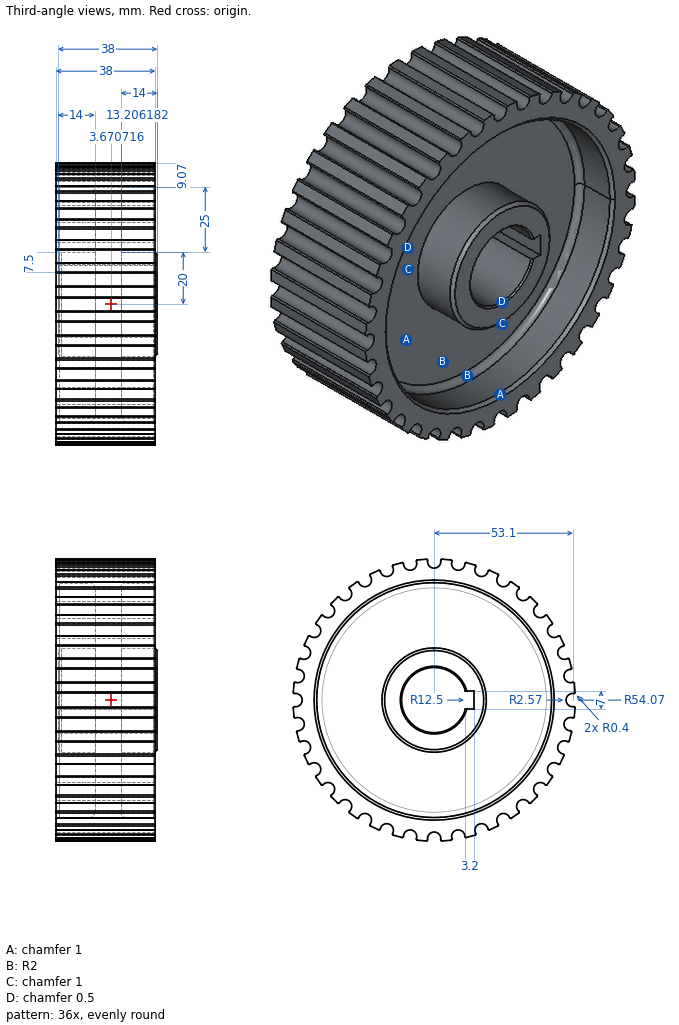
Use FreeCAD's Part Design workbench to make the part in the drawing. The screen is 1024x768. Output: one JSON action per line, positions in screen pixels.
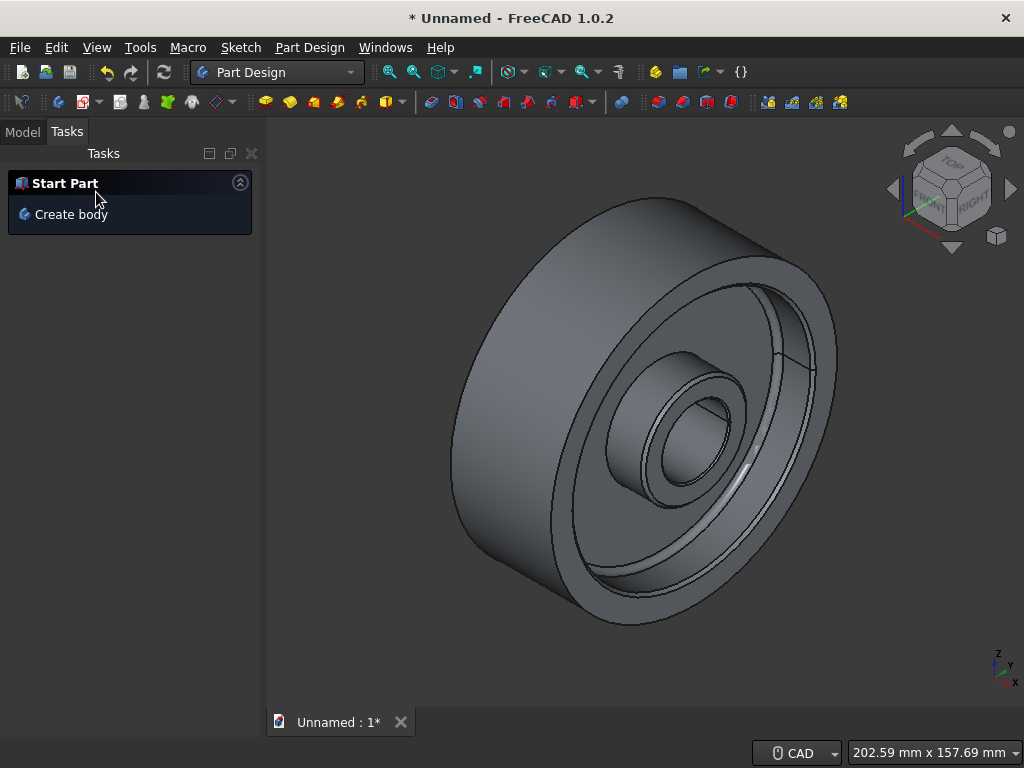
{"action": "left_click", "coordinate": [739, 416]}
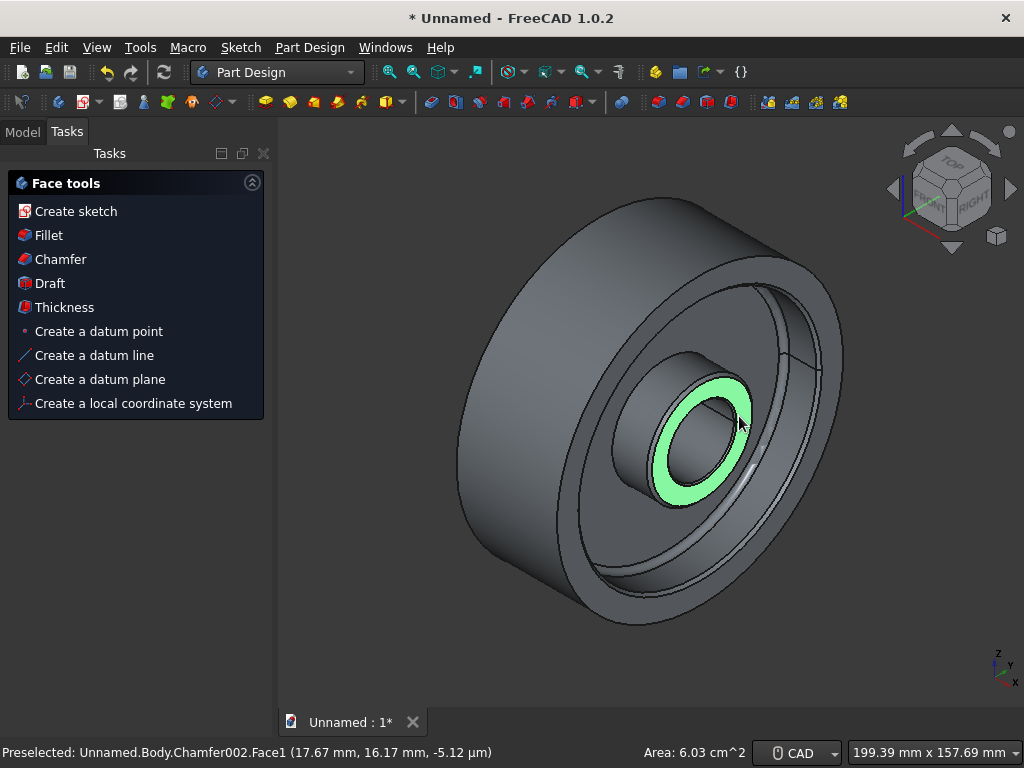
{"action": "left_click", "coordinate": [84, 102]}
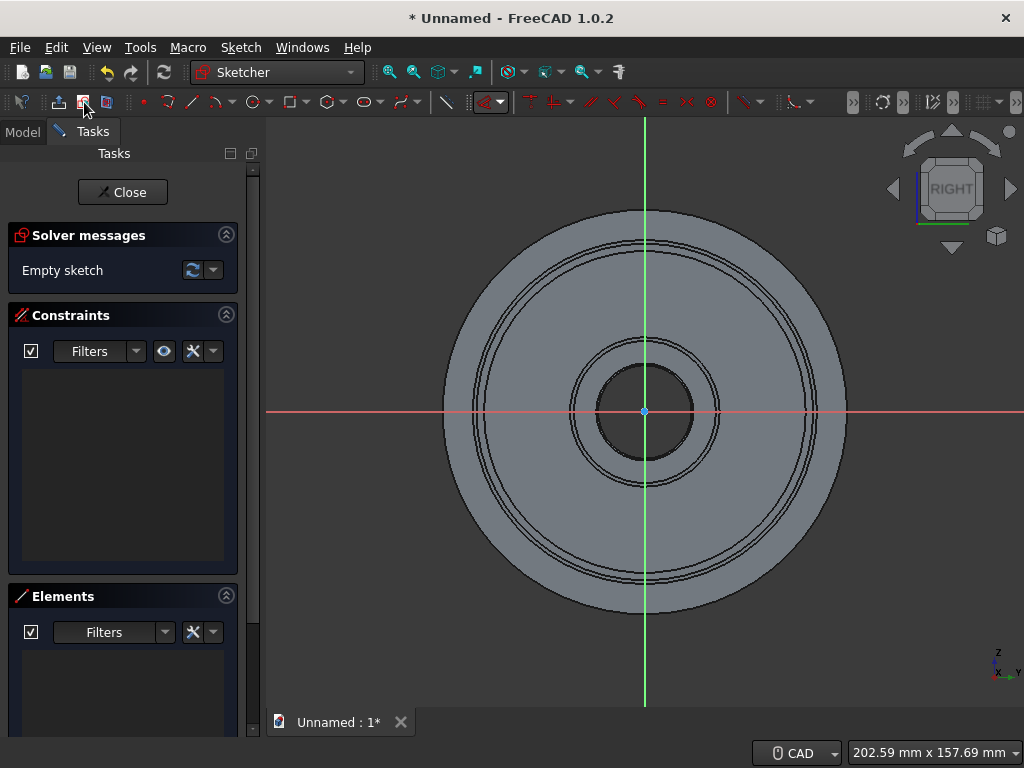
{"action": "scroll", "coordinate": [688, 412], "scroll_direction": "up", "scroll_amount": 10}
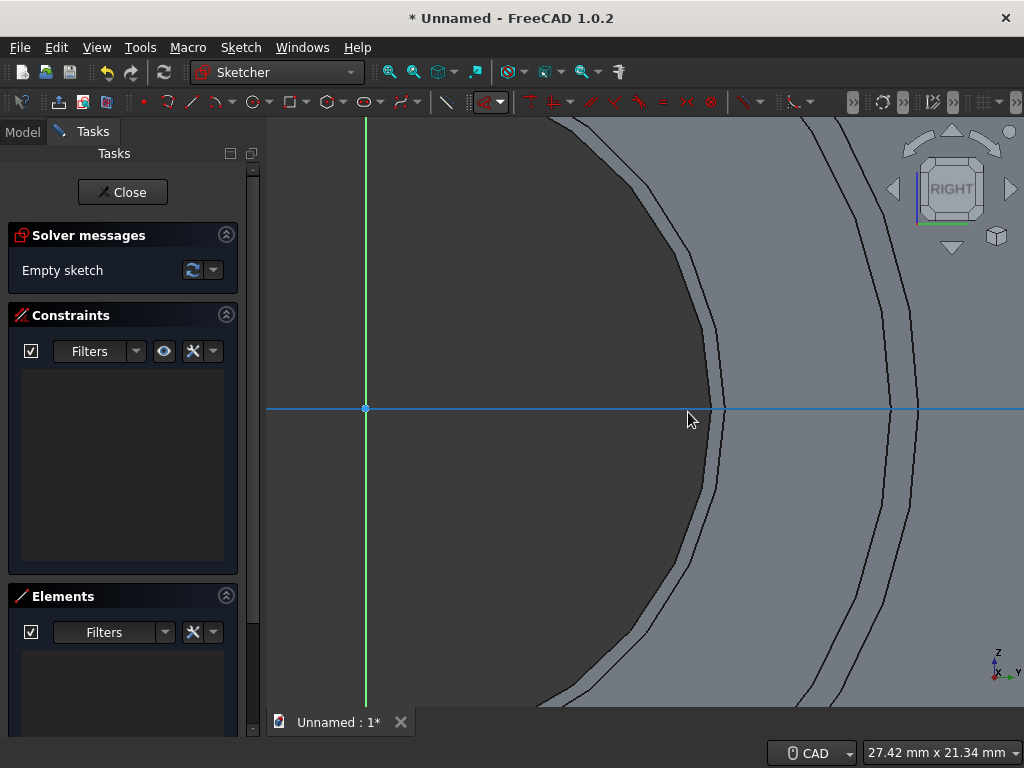
{"action": "left_click", "coordinate": [168, 102]}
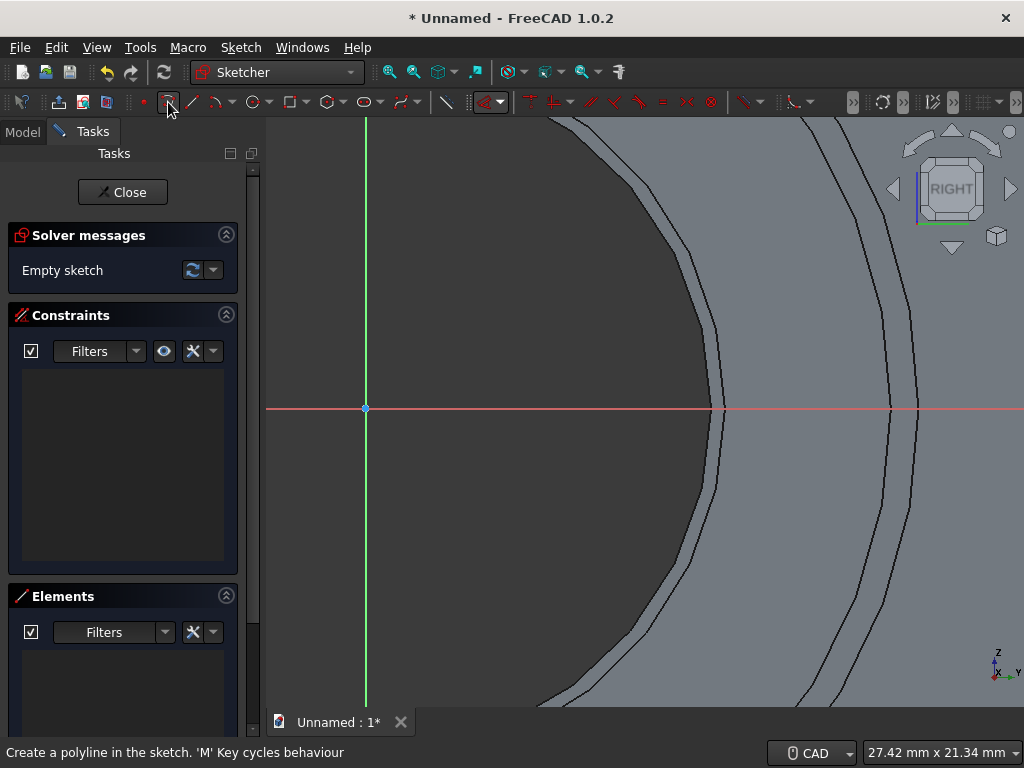
{"action": "left_click", "coordinate": [697, 506]}
{"action": "left_click", "coordinate": [786, 506]}
{"action": "left_click", "coordinate": [786, 312]}
{"action": "left_click", "coordinate": [697, 312]}
{"action": "right_click", "coordinate": [697, 312]}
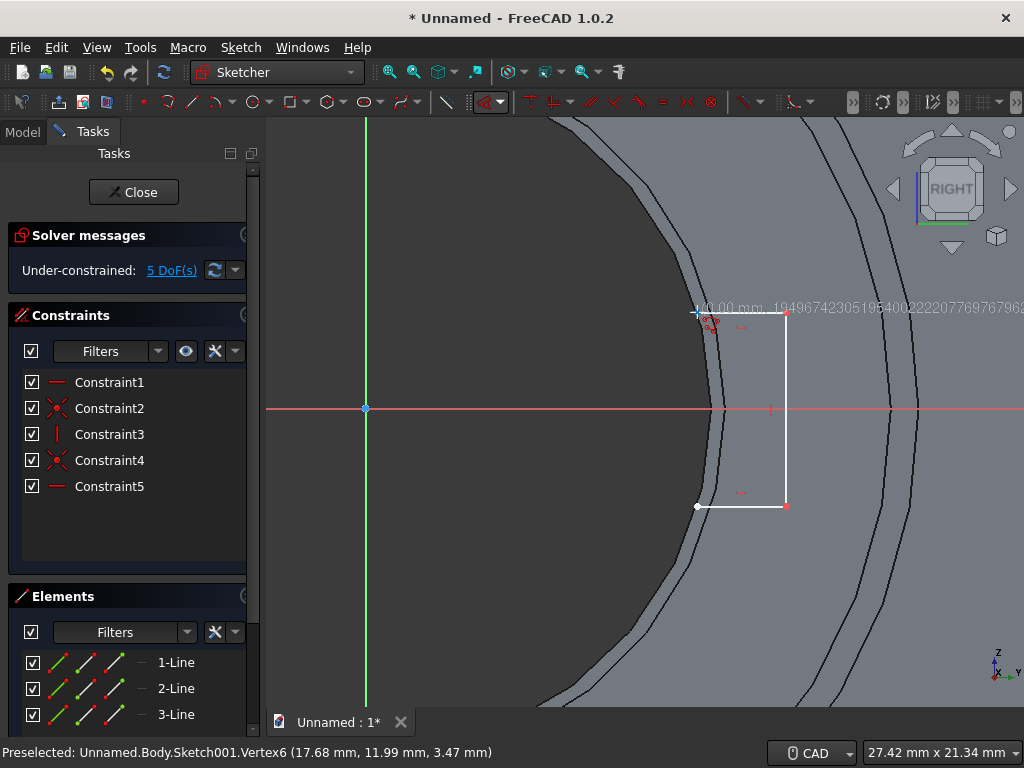
{"action": "key", "text": "g 3 a"}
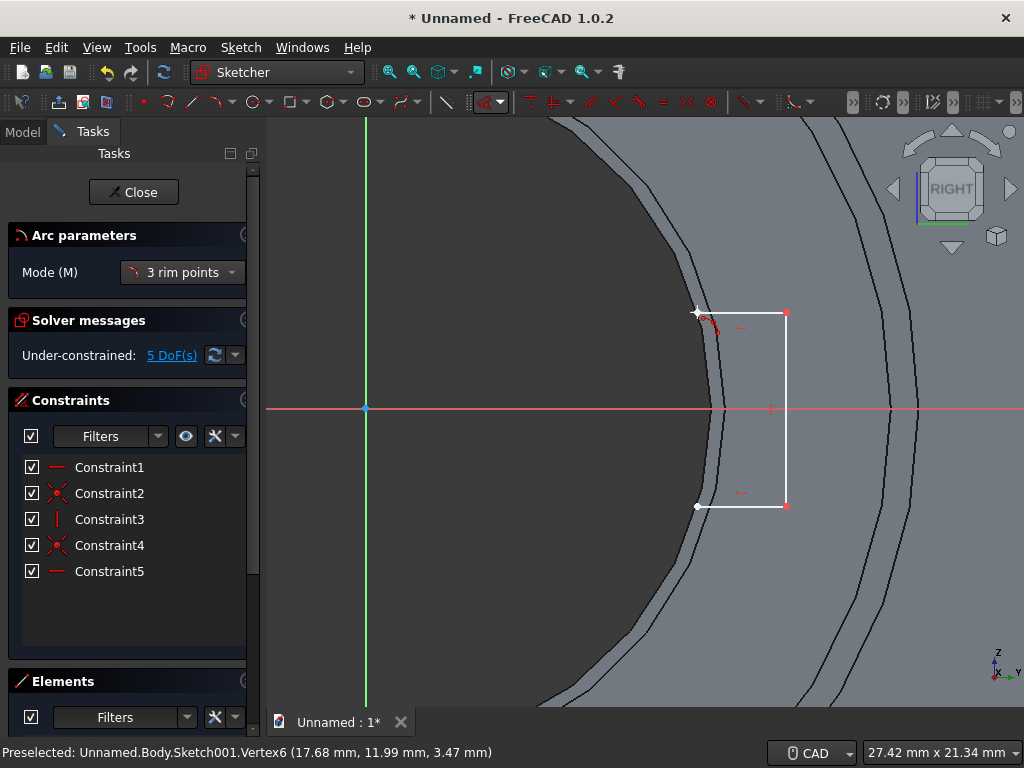
{"action": "left_click", "coordinate": [697, 313]}
{"action": "left_click", "coordinate": [697, 507]}
{"action": "left_click", "coordinate": [711, 428]}
{"action": "key", "text": "Escape"}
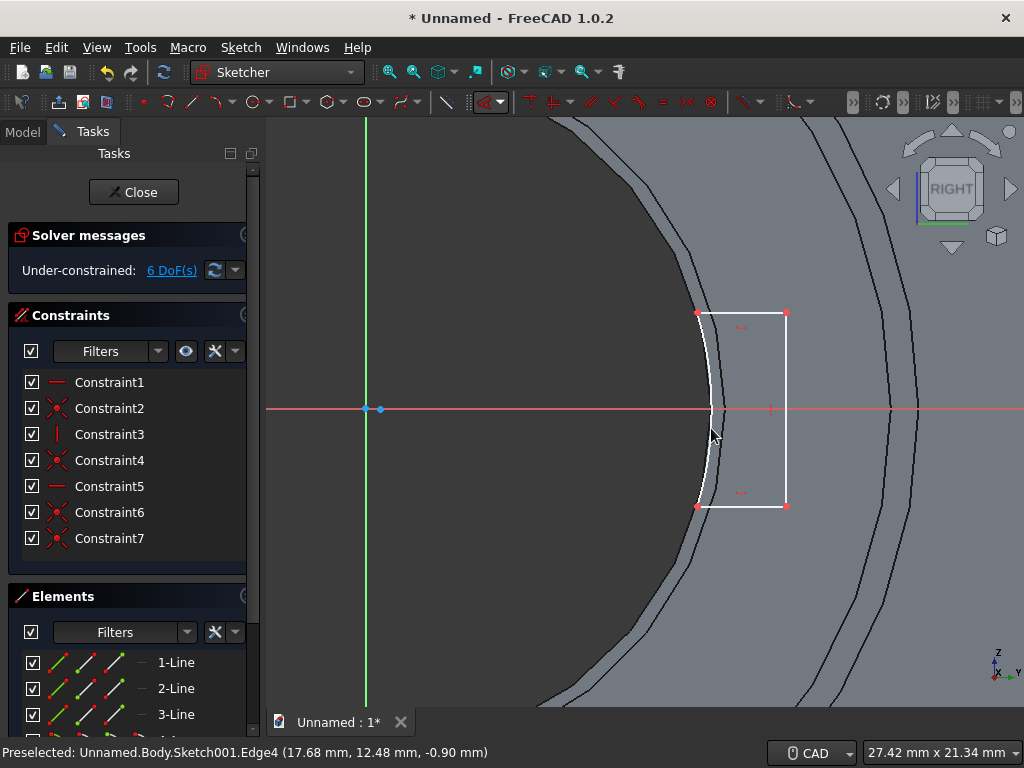
{"action": "left_click_drag", "start_coordinate": [356, 399], "coordinate": [391, 420]}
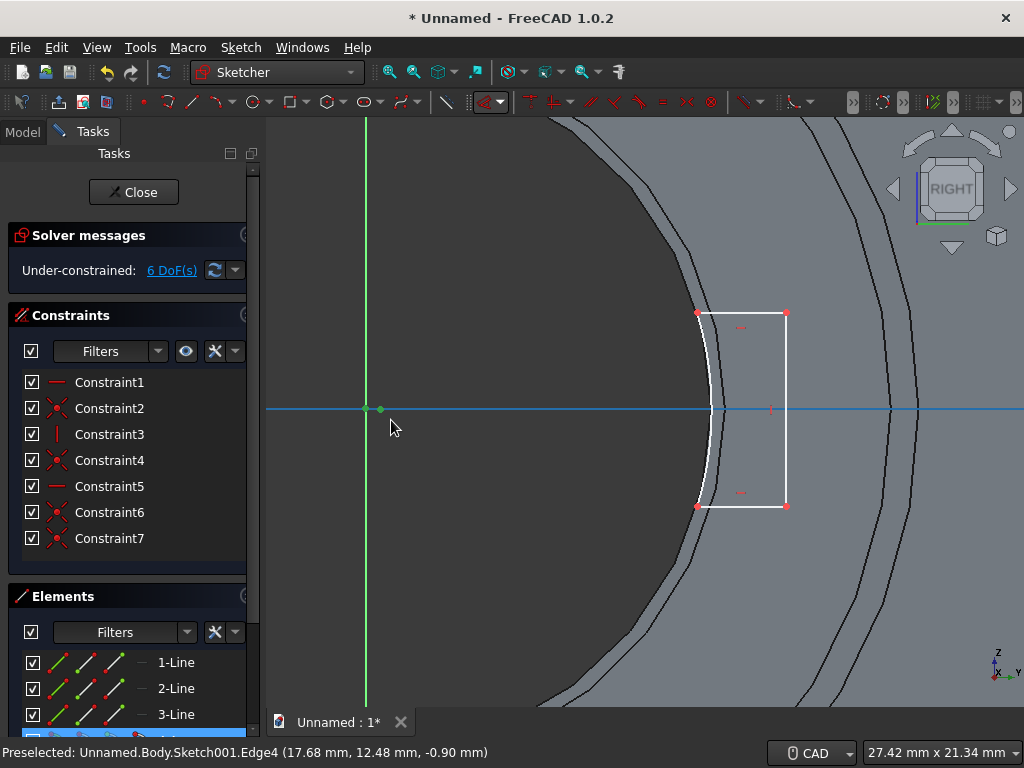
{"action": "key", "text": "c"}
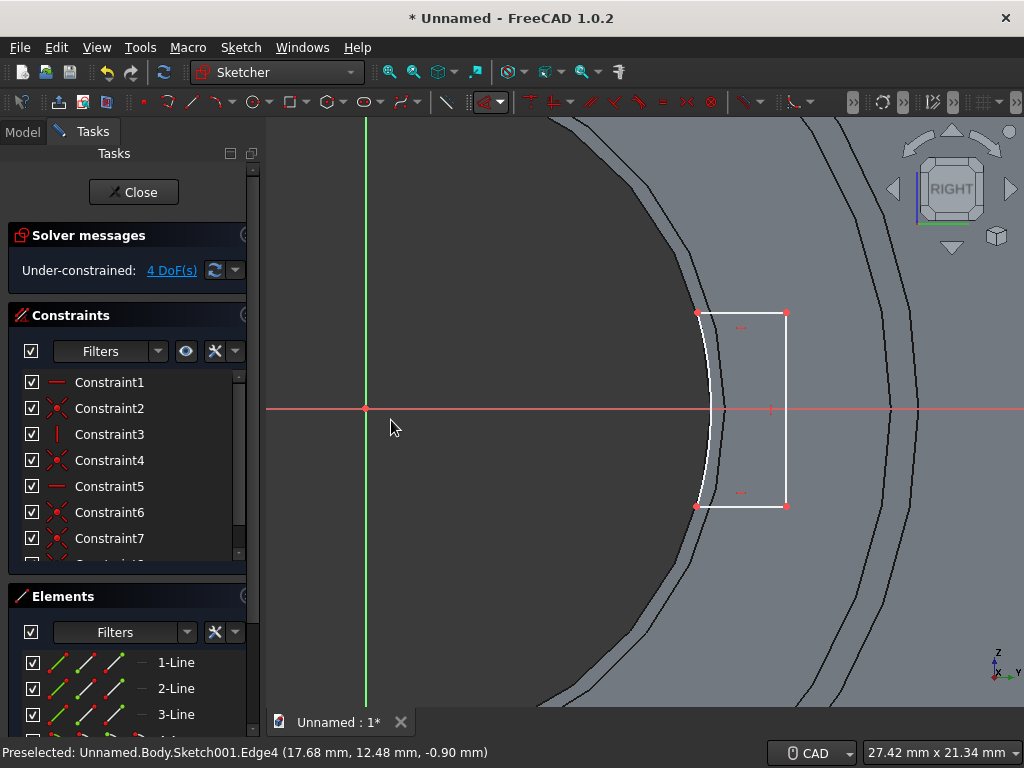
{"action": "left_click", "coordinate": [709, 449]}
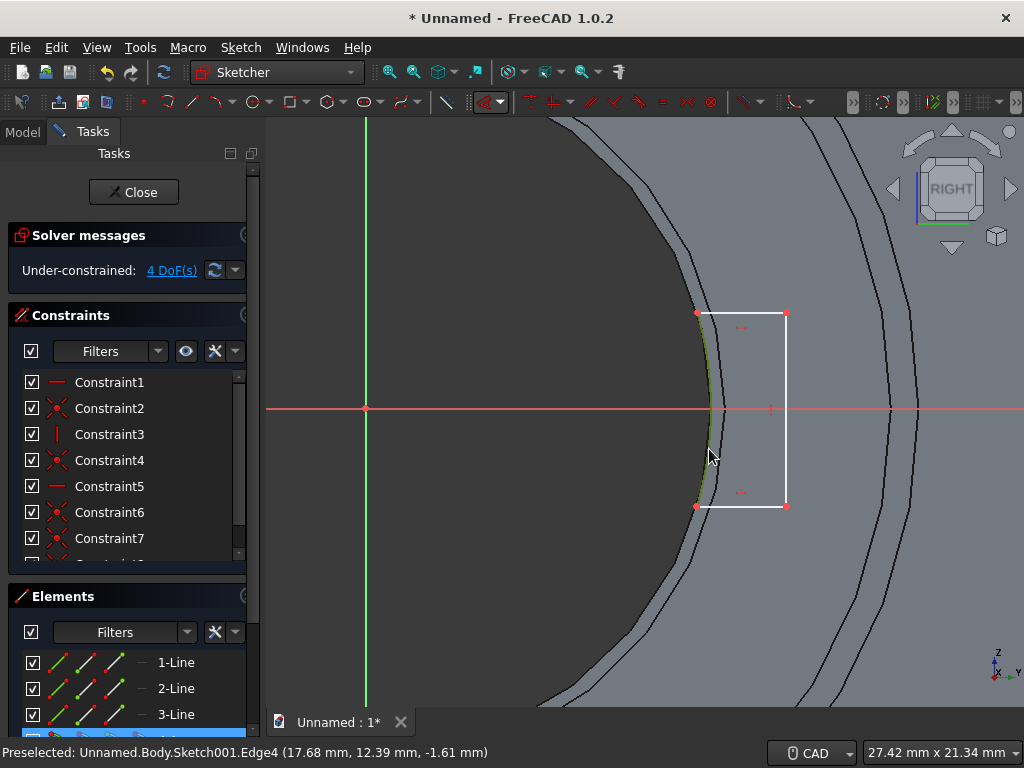
{"action": "key", "text": "k r"}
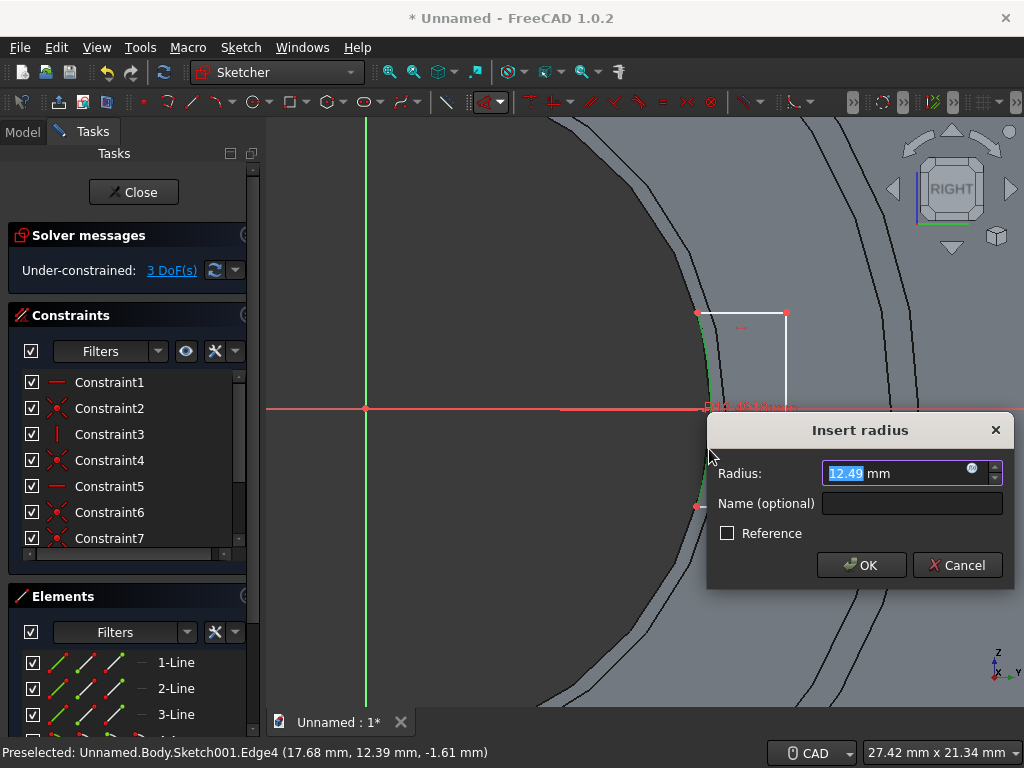
{"action": "type", "text": "12.5"}
{"action": "key", "text": "Return"}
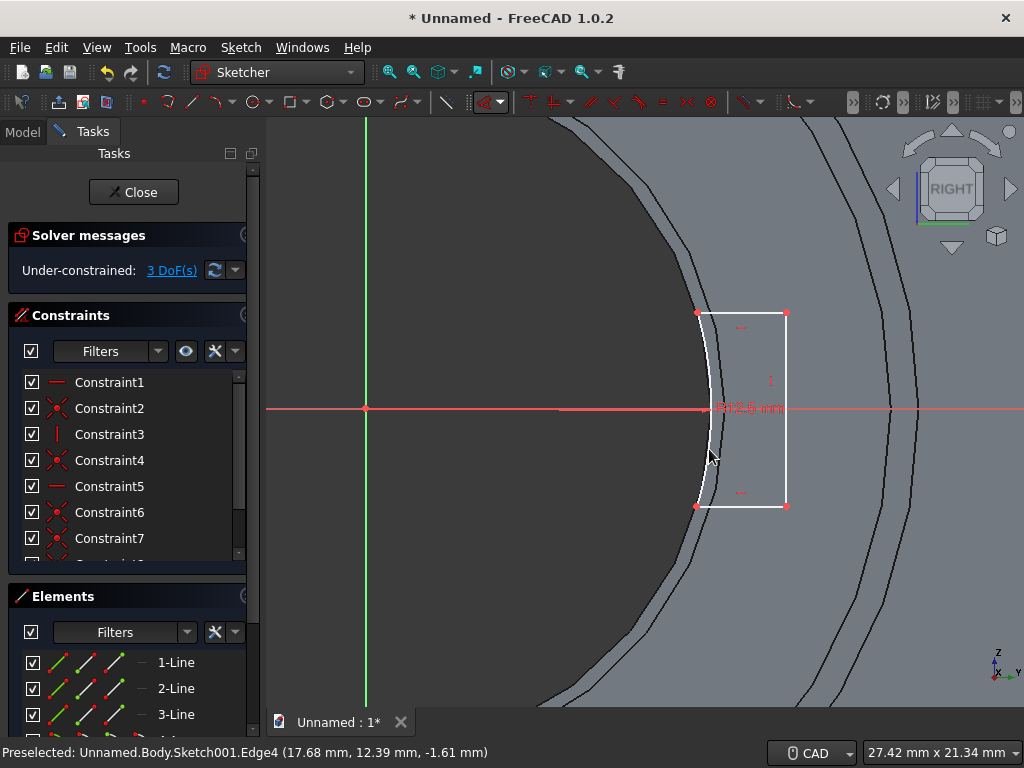
{"action": "left_click", "coordinate": [786, 449]}